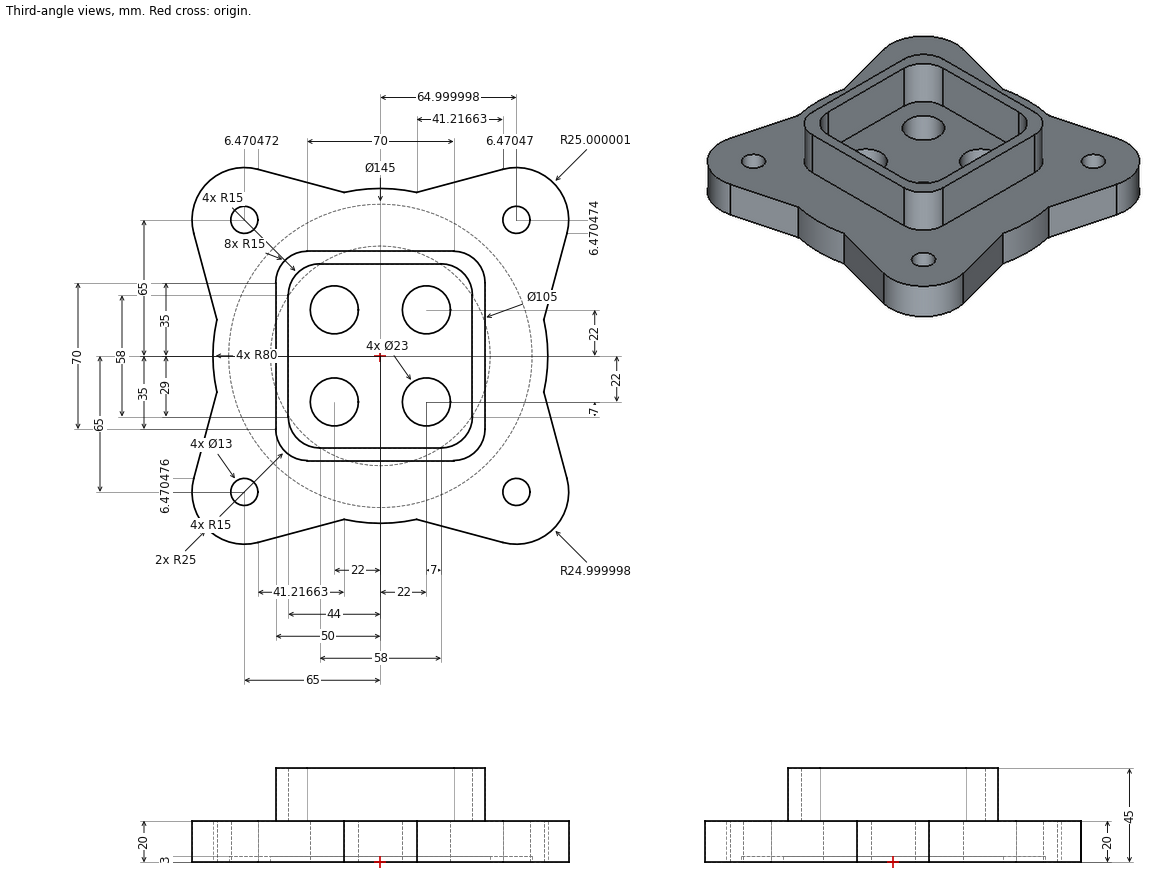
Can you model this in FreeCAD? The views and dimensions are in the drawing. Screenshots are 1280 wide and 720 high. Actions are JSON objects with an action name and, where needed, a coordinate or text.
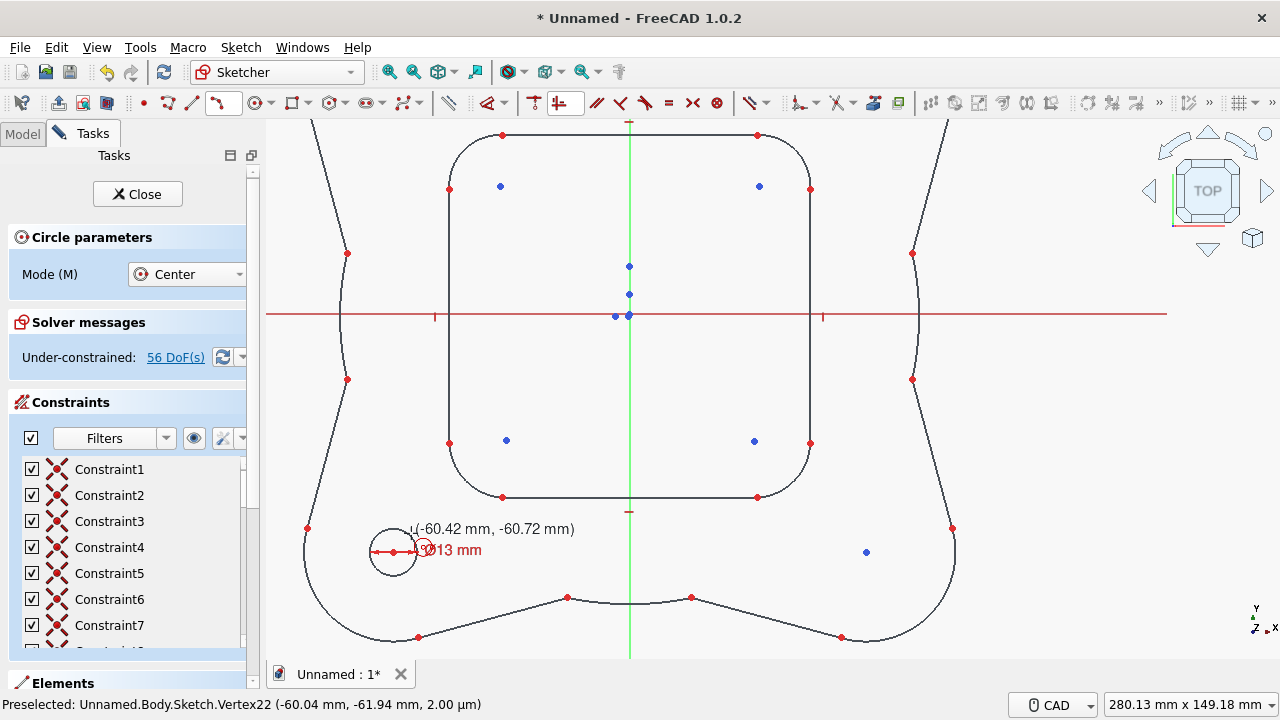
{"action": "left_click", "coordinate": [865, 549]}
{"action": "mouse_move", "coordinate": [882, 533]}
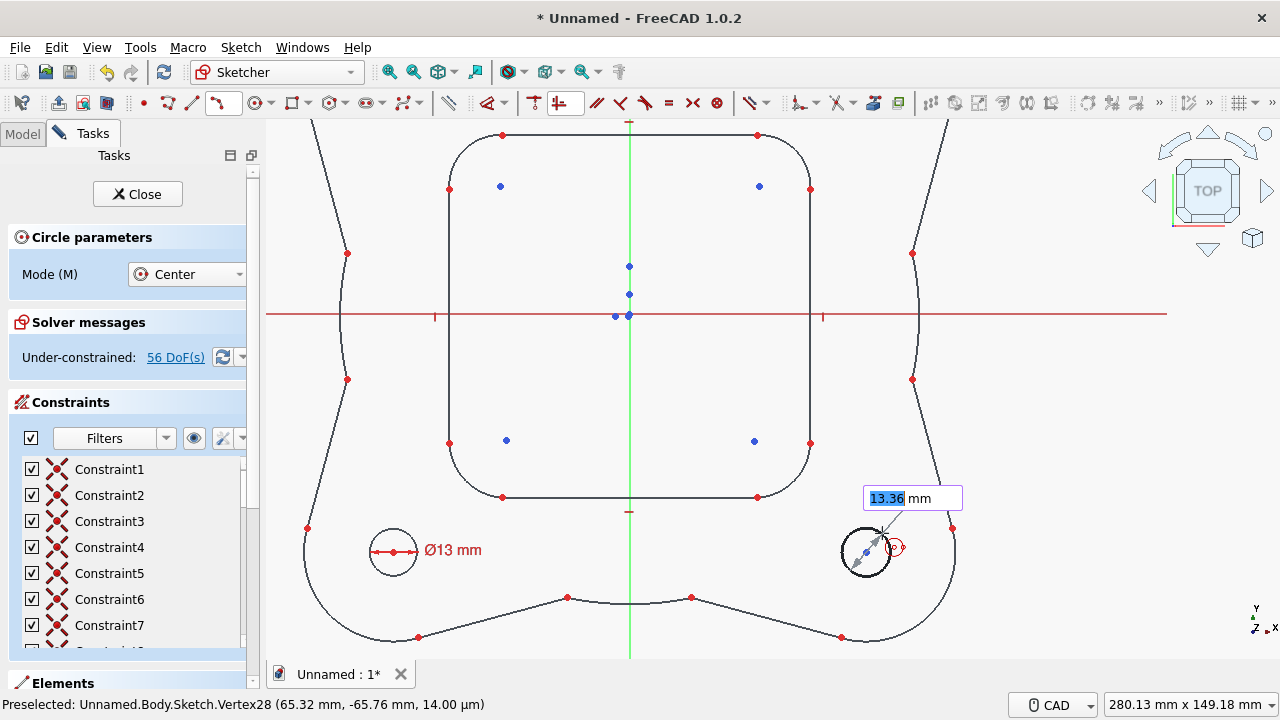
{"action": "type", "text": "13"}
{"action": "key", "text": "Return"}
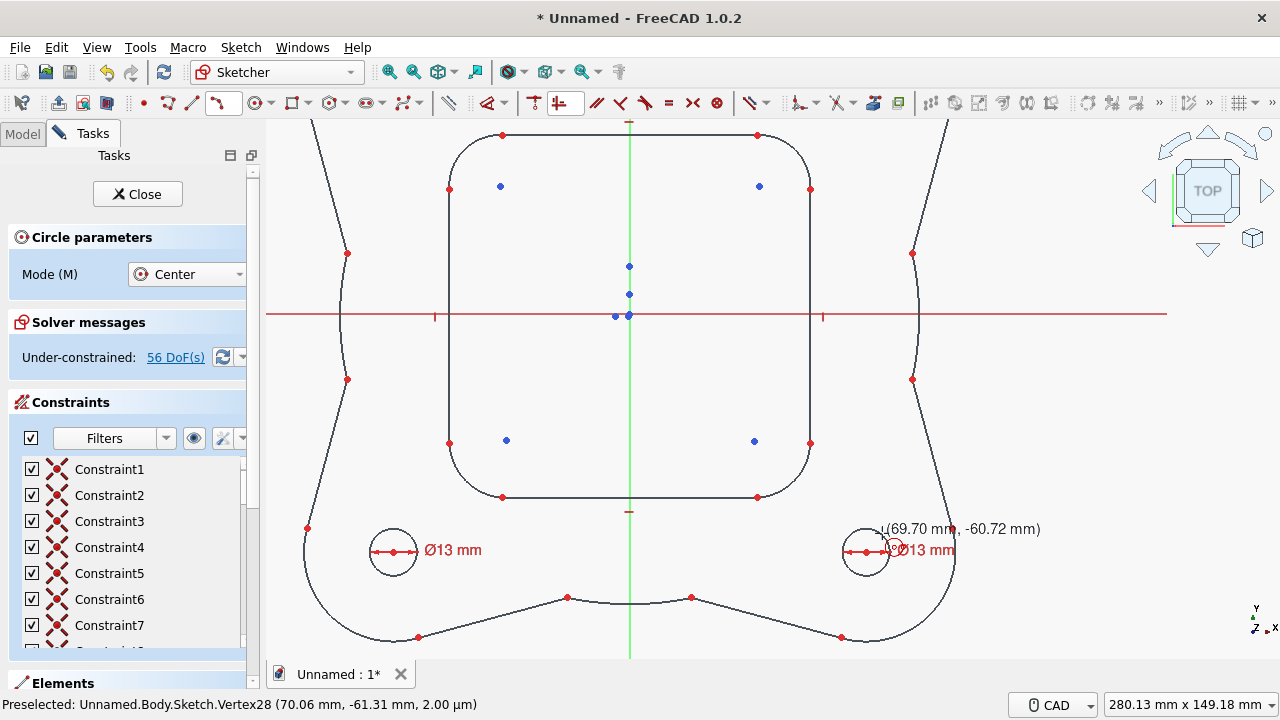
{"action": "scroll", "coordinate": [795, 480], "scroll_direction": "down", "scroll_amount": 3}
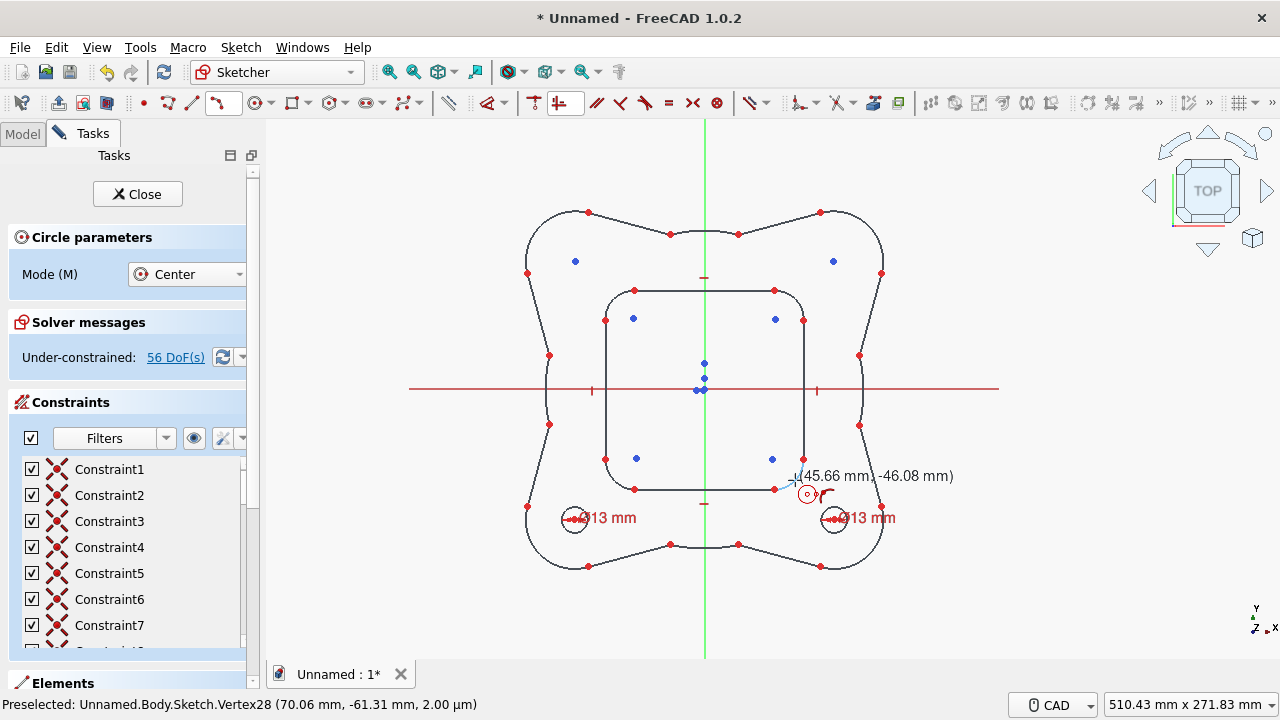
{"action": "scroll", "coordinate": [575, 260], "scroll_direction": "up", "scroll_amount": 3}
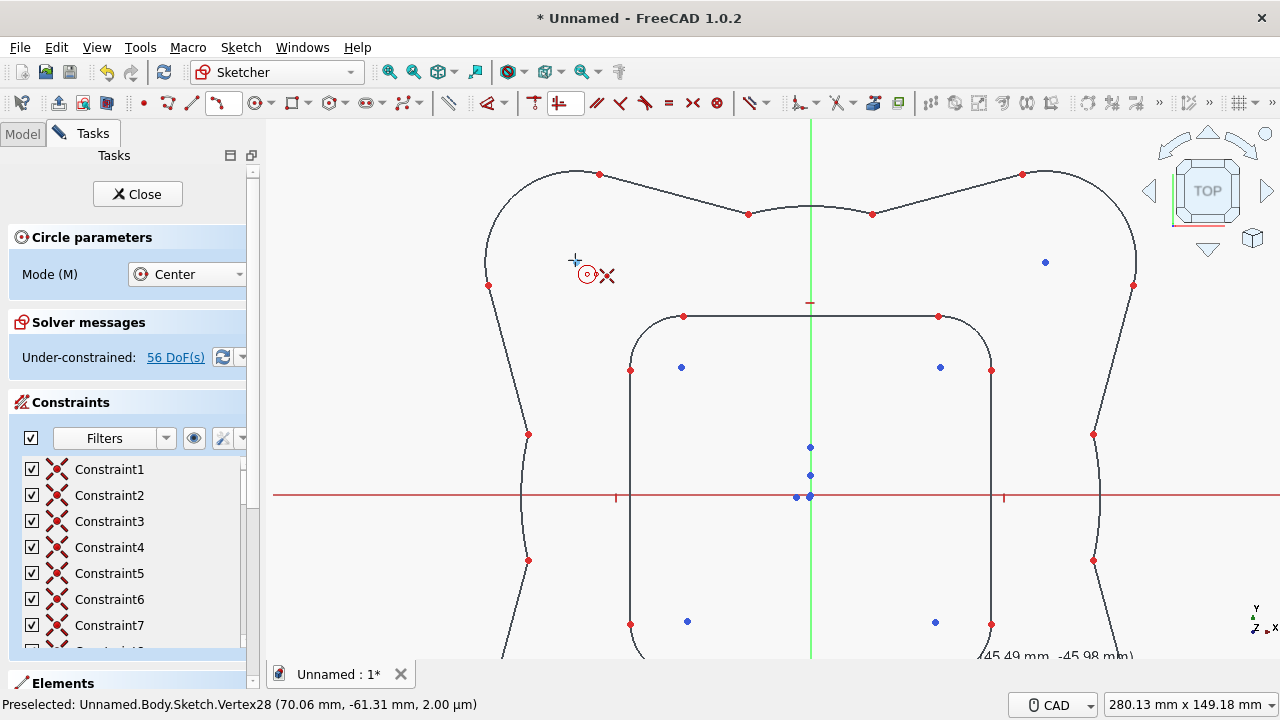
{"action": "left_click", "coordinate": [575, 260]}
{"action": "mouse_move", "coordinate": [592, 243]}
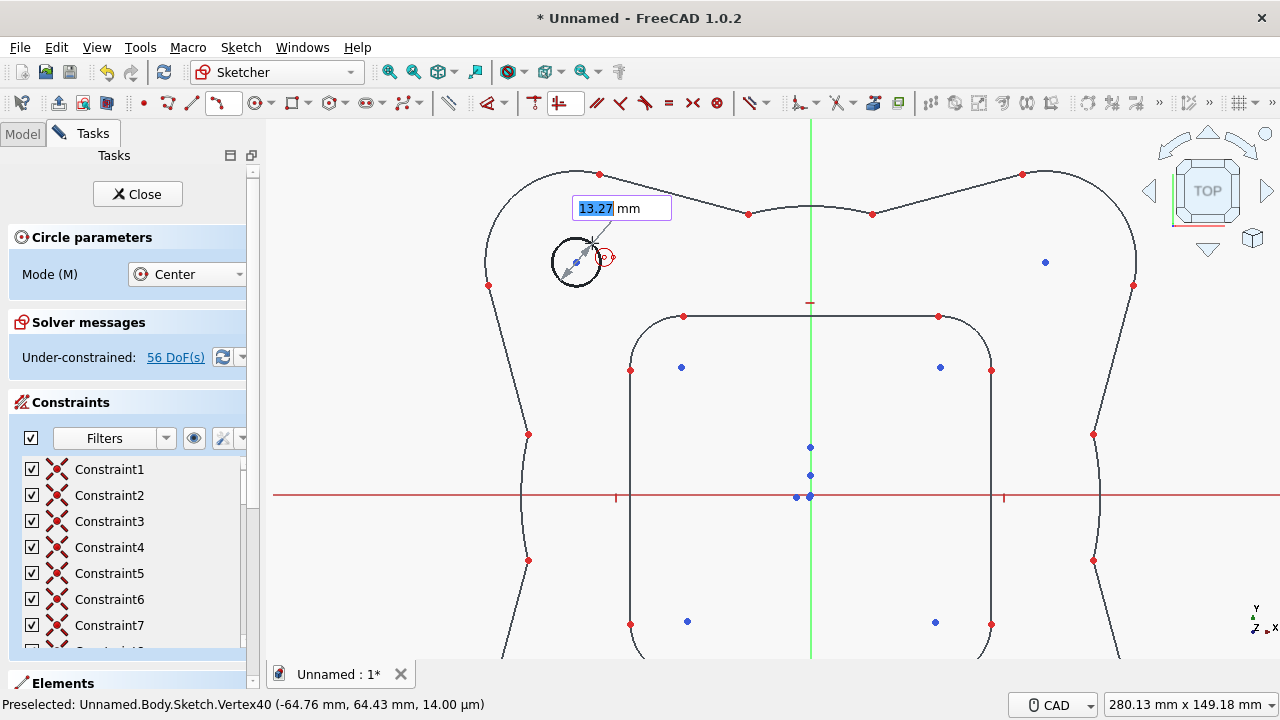
{"action": "type", "text": "13"}
{"action": "key", "text": "Return"}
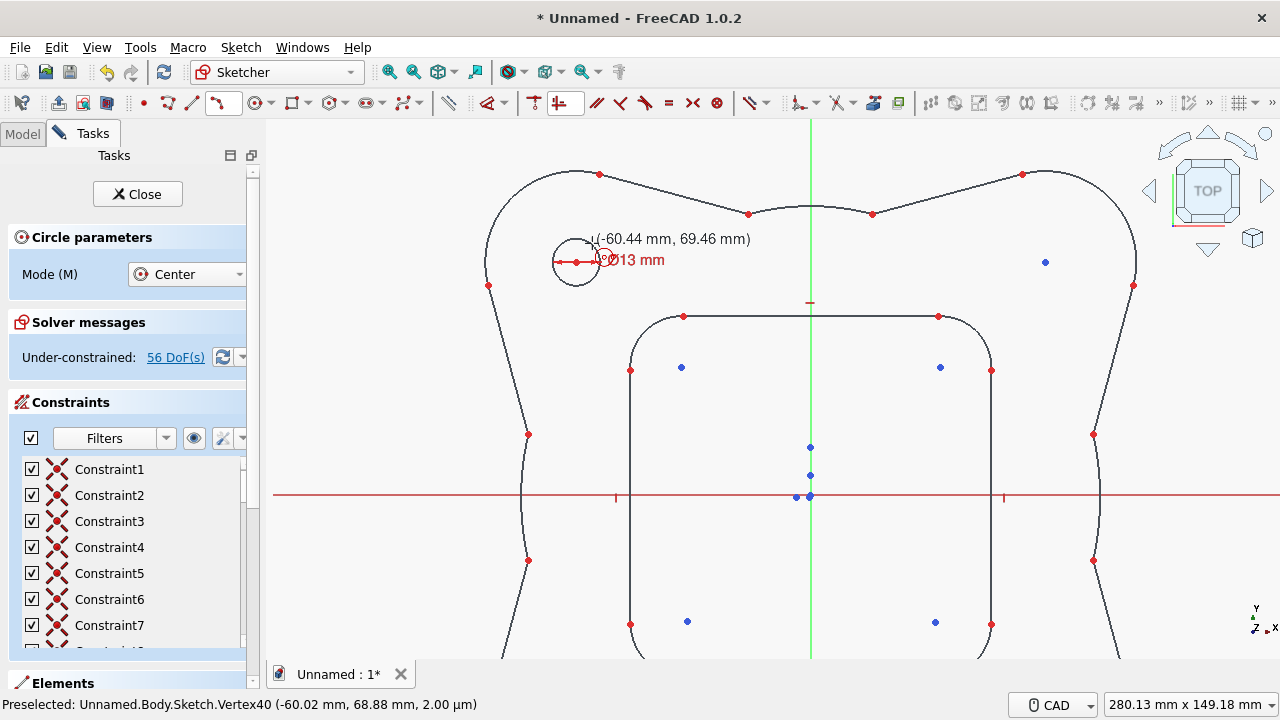
{"action": "left_click", "coordinate": [1046, 260]}
{"action": "mouse_move", "coordinate": [1063, 243]}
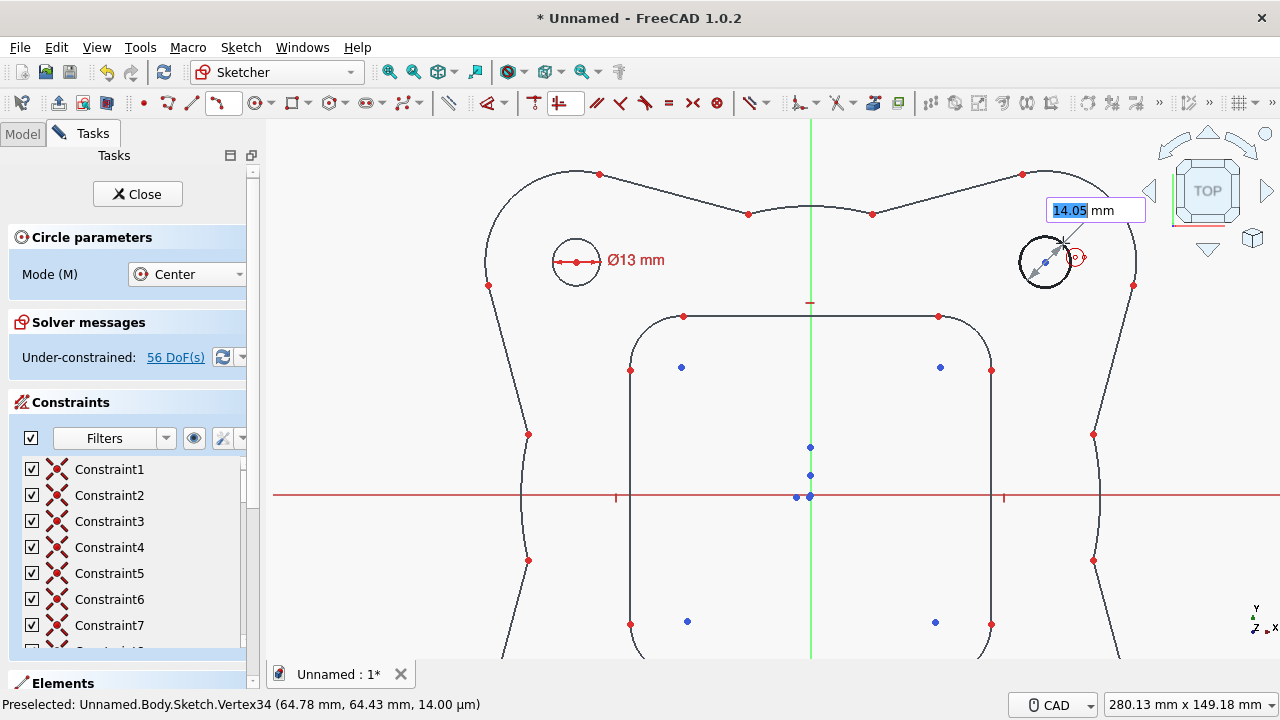
{"action": "type", "text": "13"}
{"action": "key", "text": "Return"}
{"action": "key", "text": "Escape"}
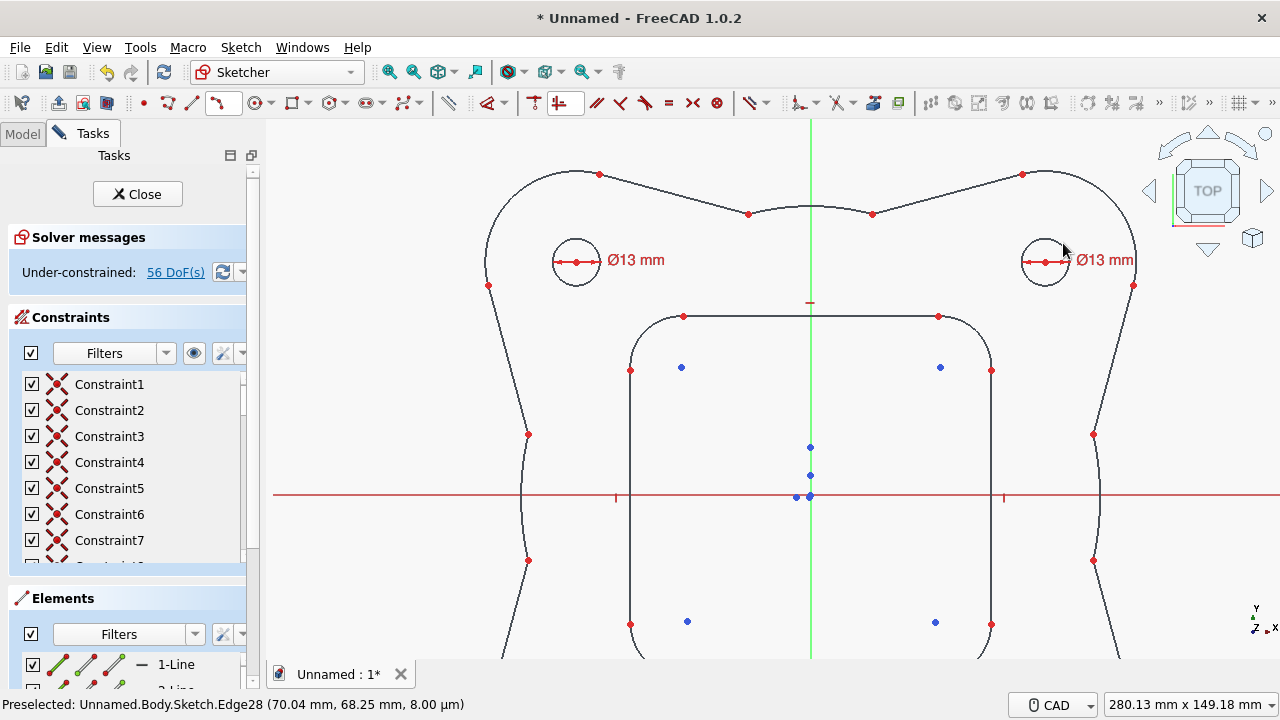
{"action": "left_click", "coordinate": [500, 330]}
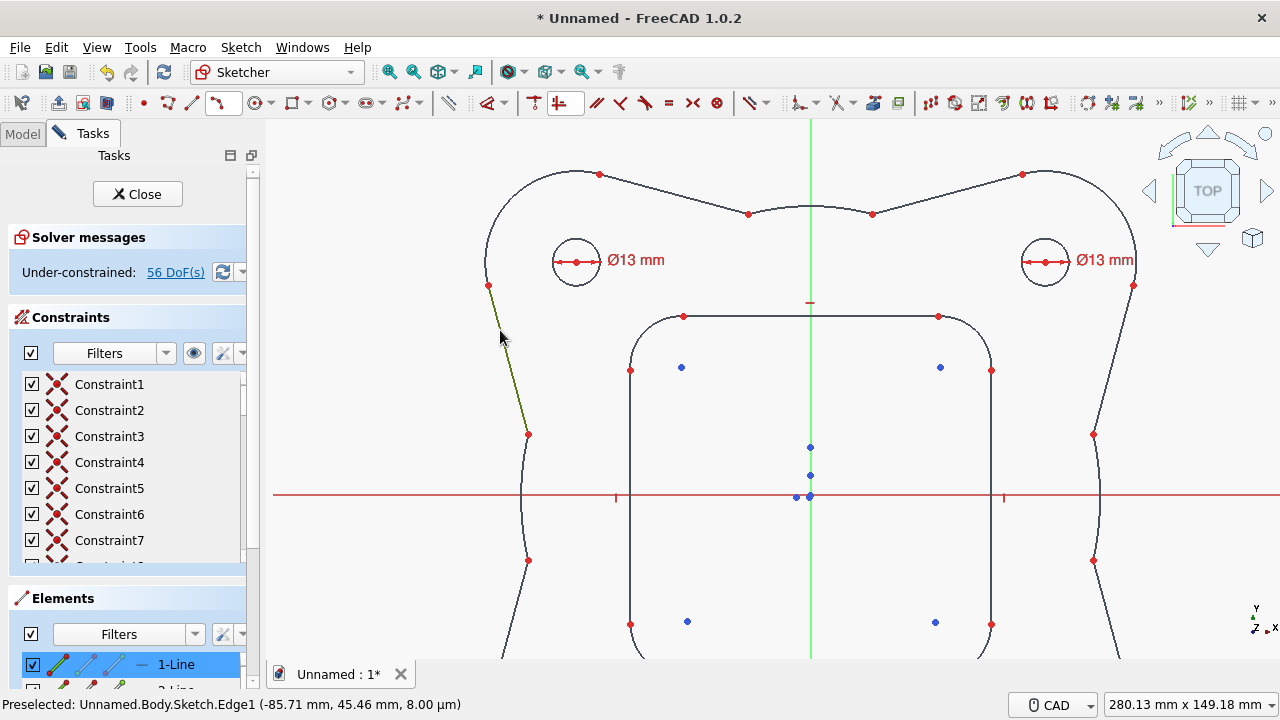
{"action": "left_click", "coordinate": [544, 177]}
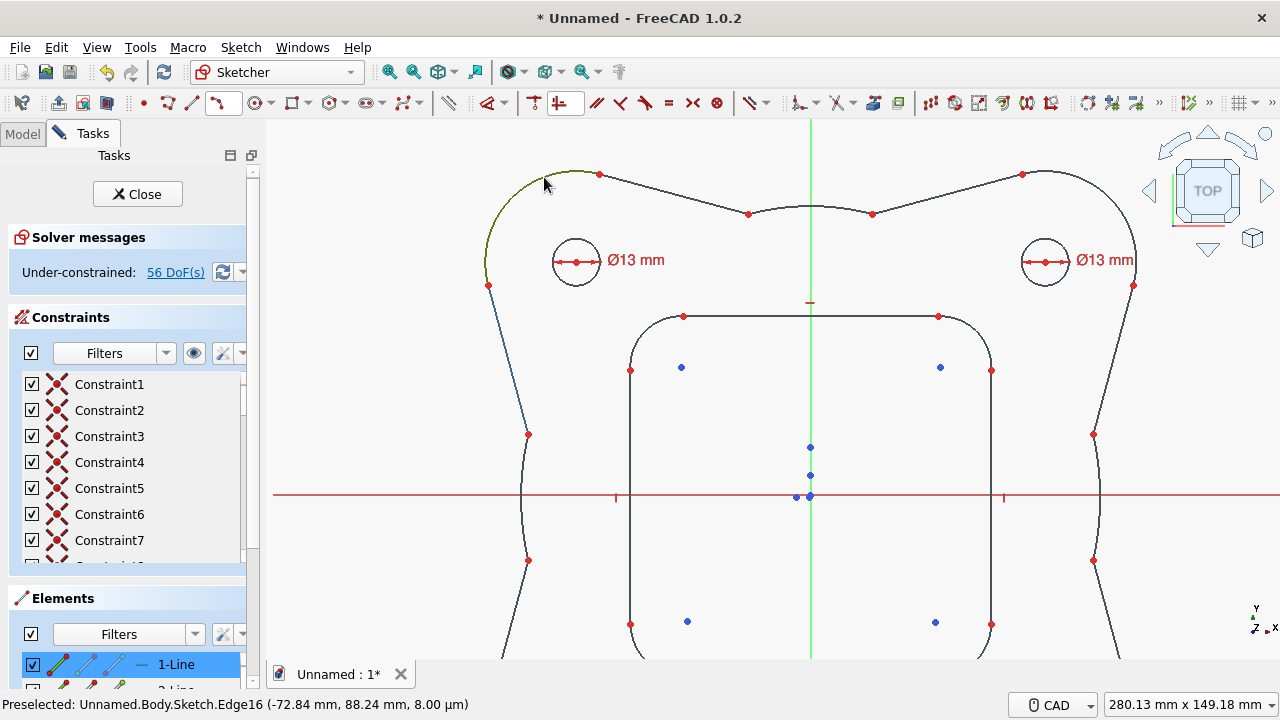
{"action": "left_click", "coordinate": [646, 104]}